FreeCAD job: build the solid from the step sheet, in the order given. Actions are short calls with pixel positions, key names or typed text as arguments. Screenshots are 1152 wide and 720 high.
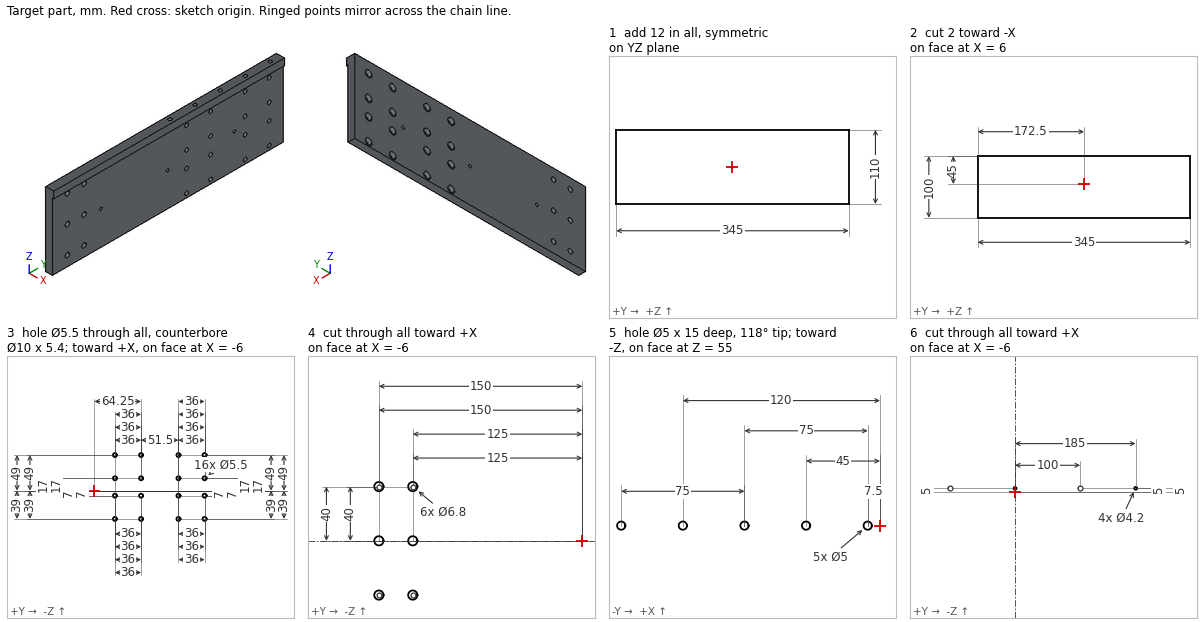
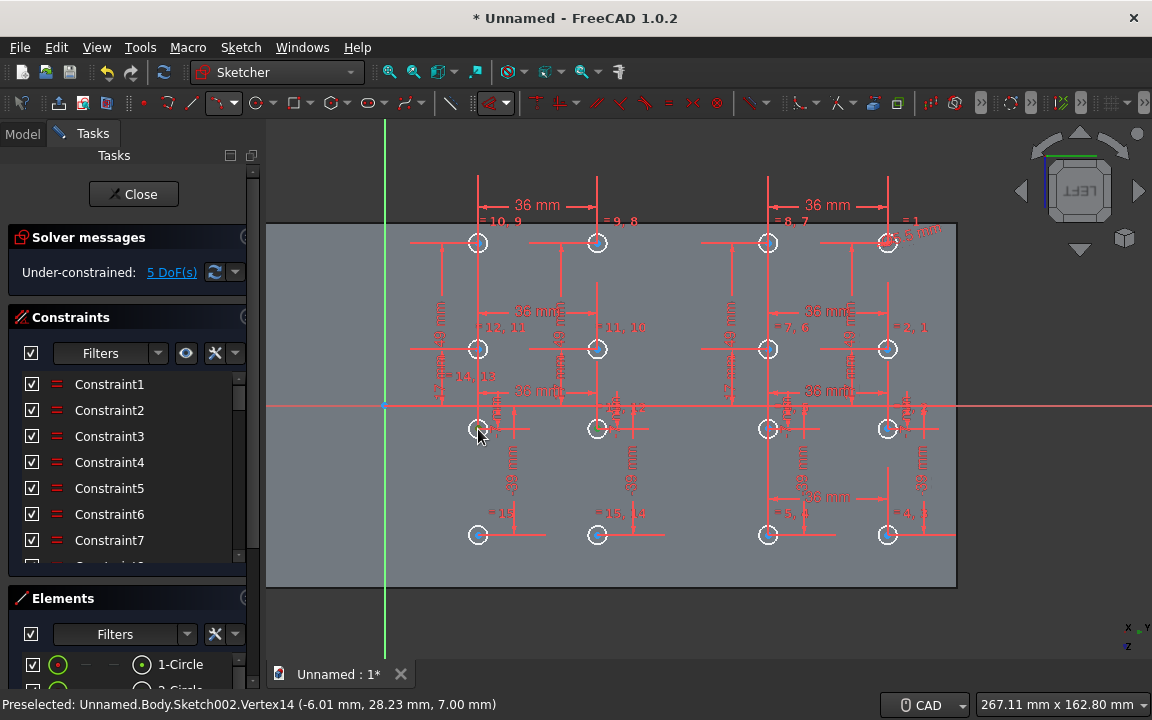
click(508, 104)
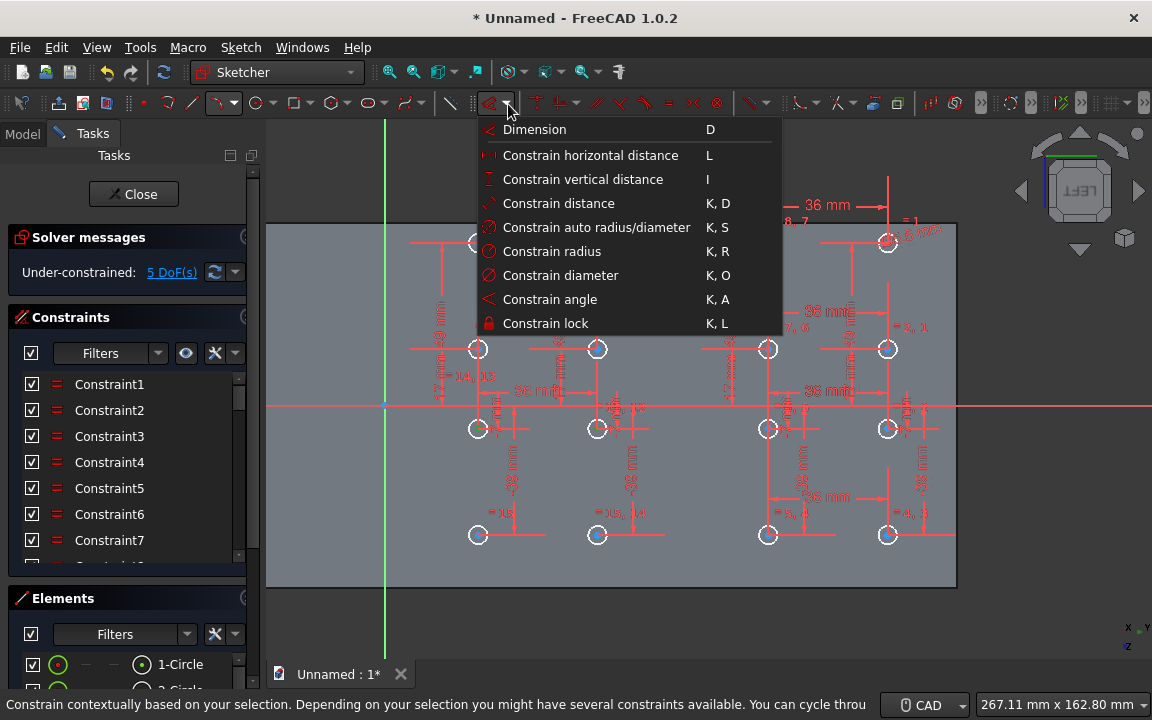
click(630, 155)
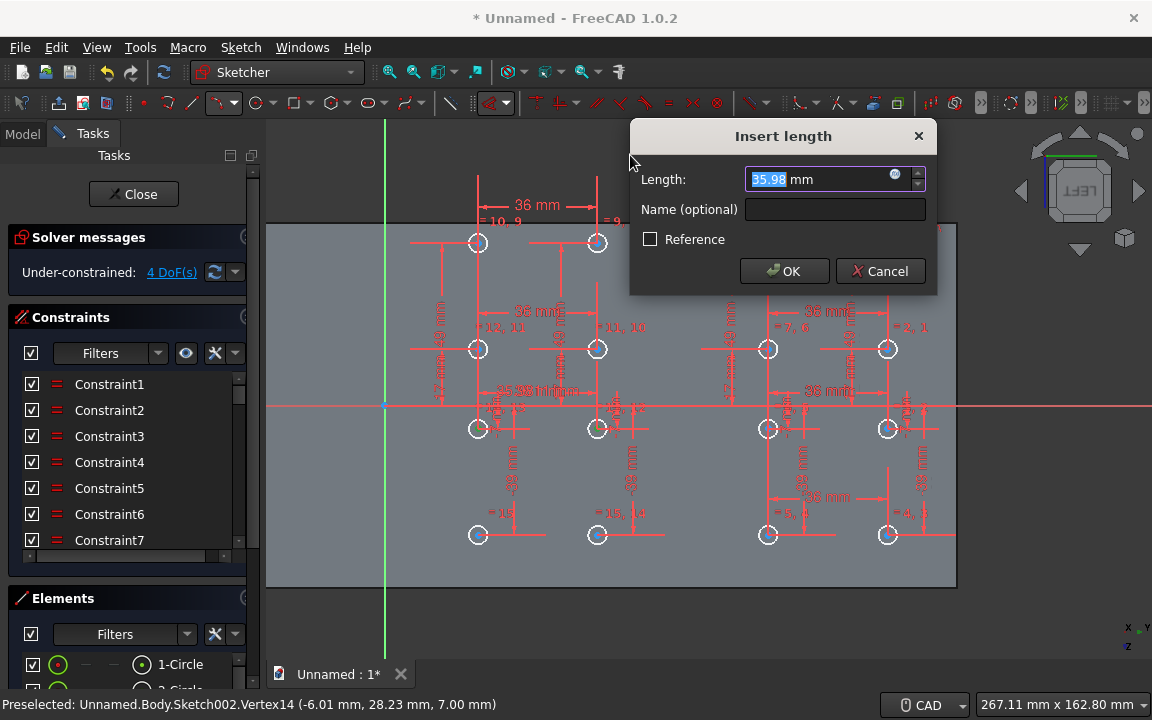
text(36)
key(Return)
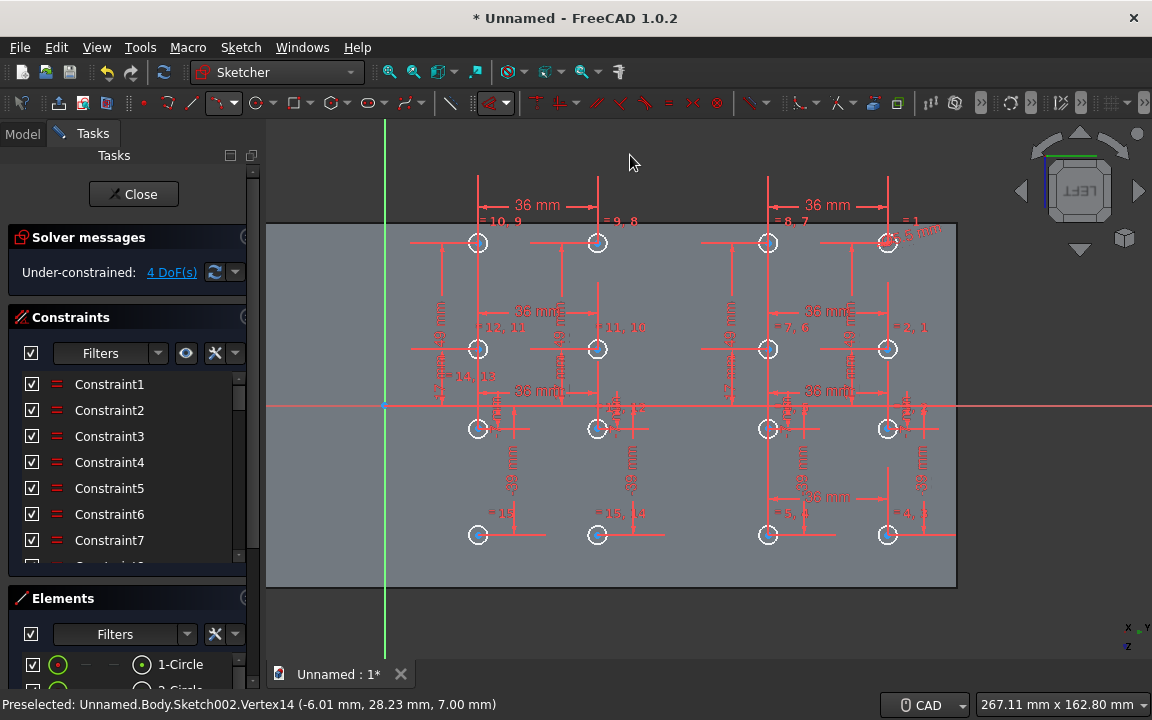
click(478, 429)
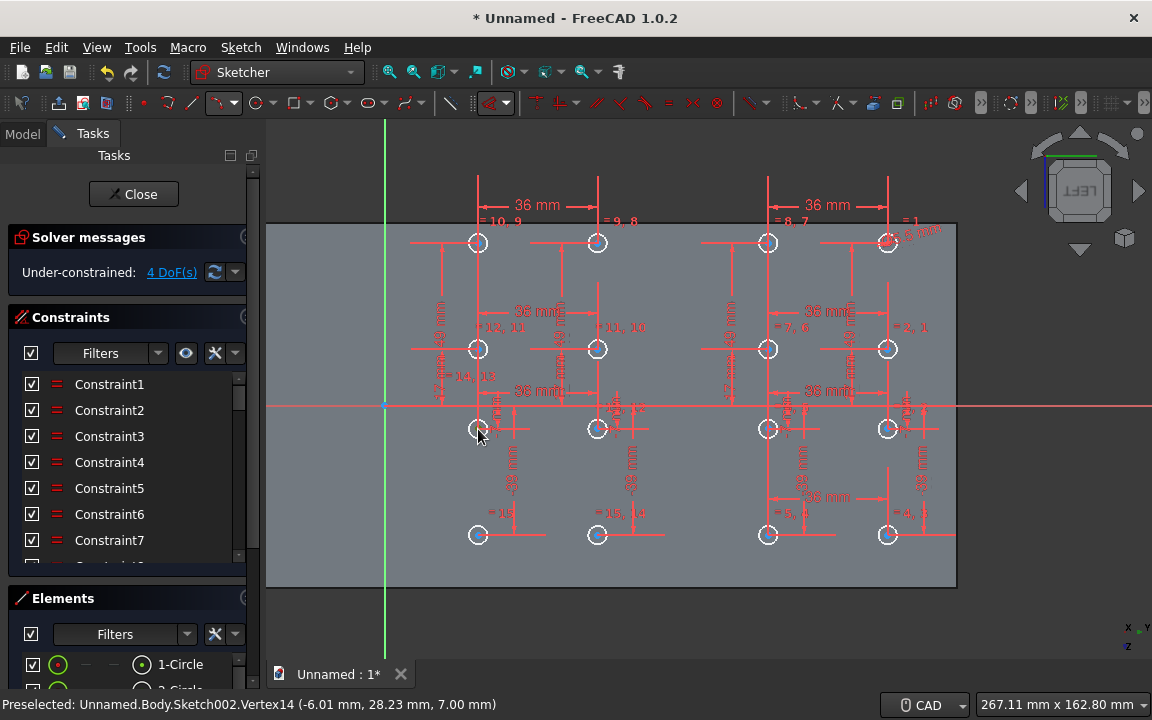
click(598, 535)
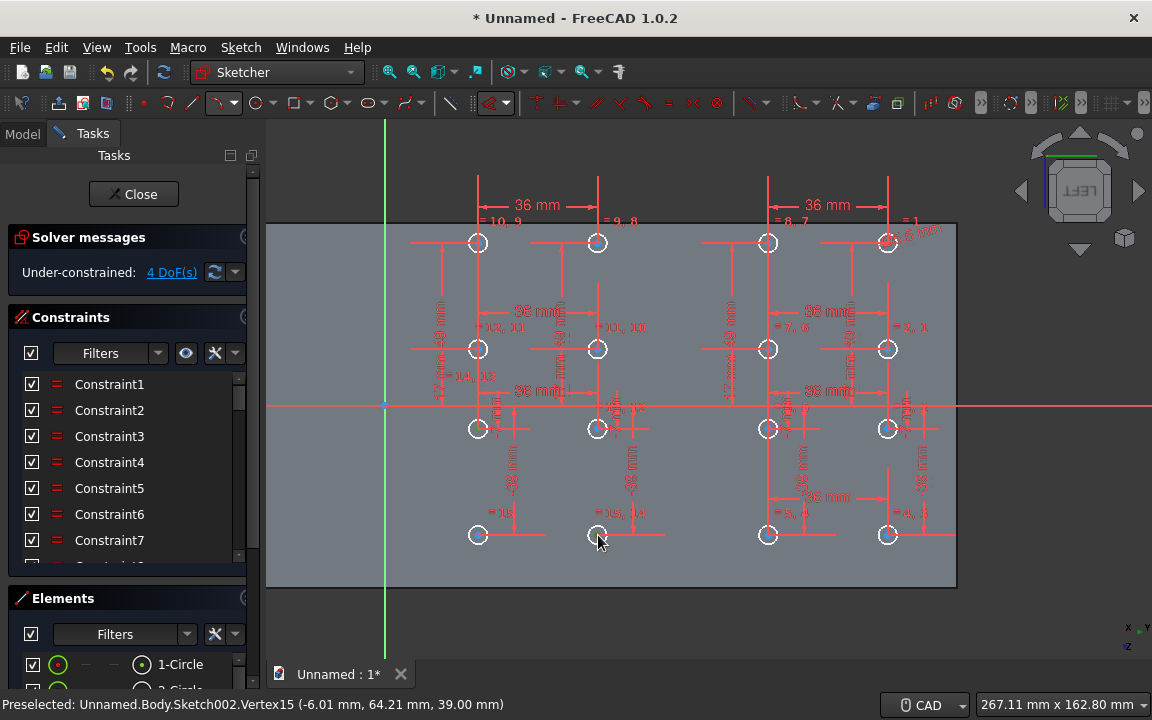
click(508, 104)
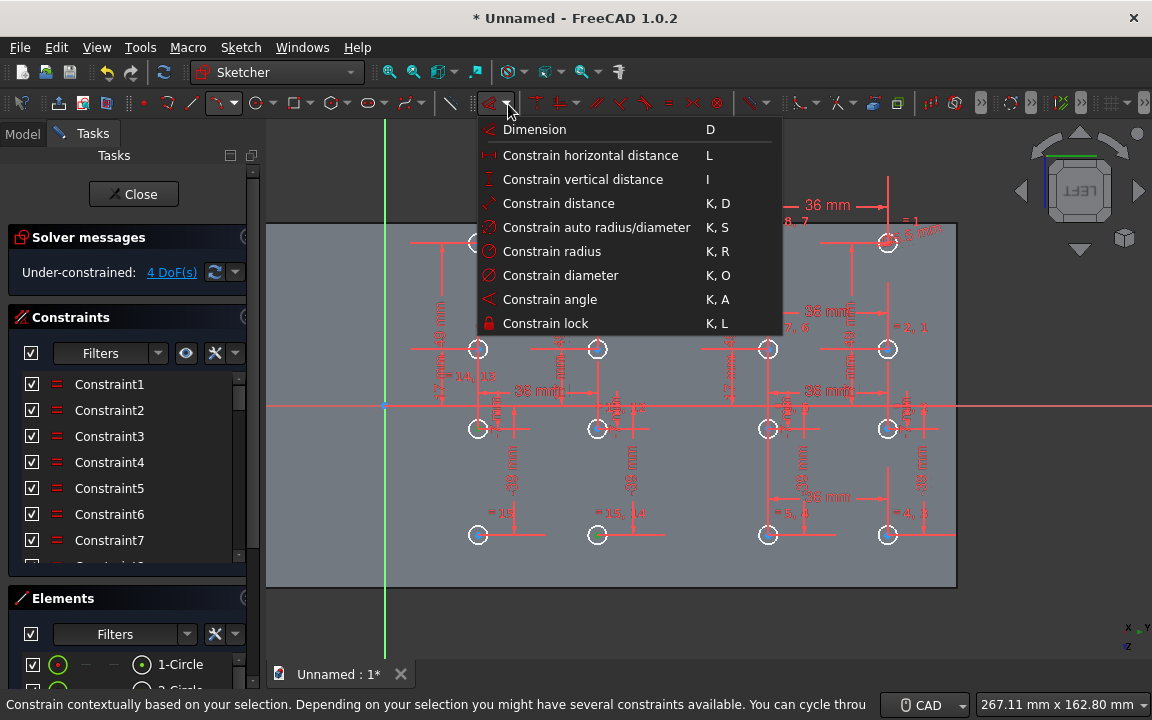
click(630, 155)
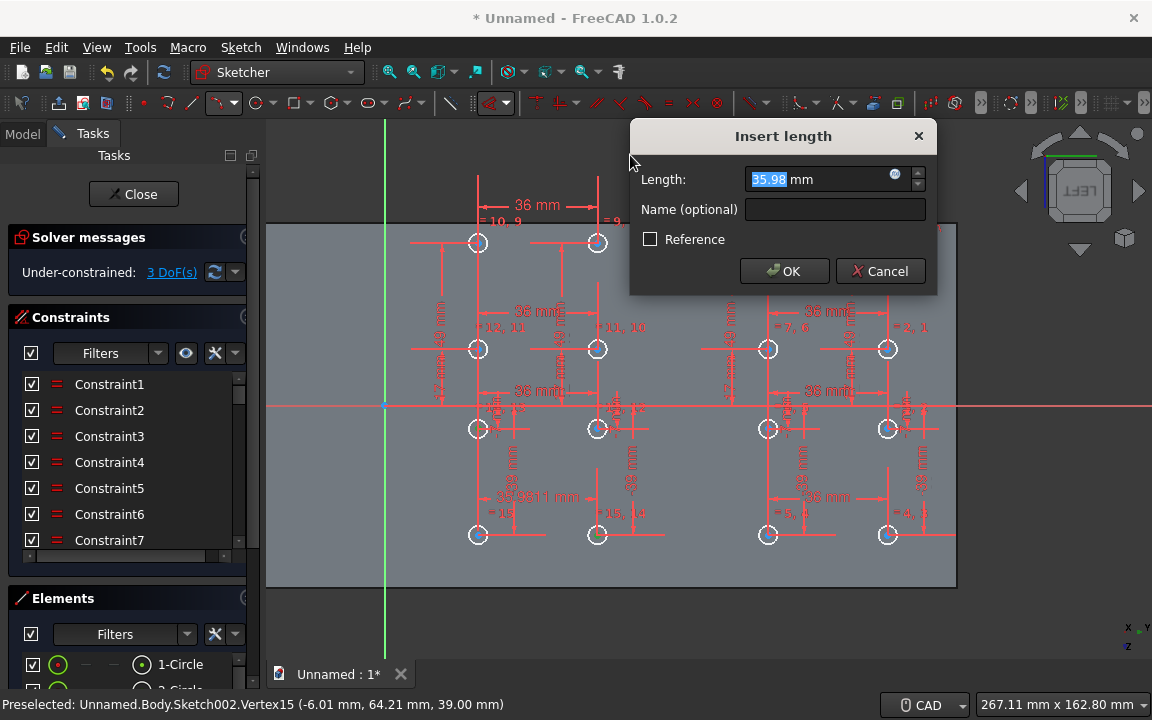
text(36)
key(Return)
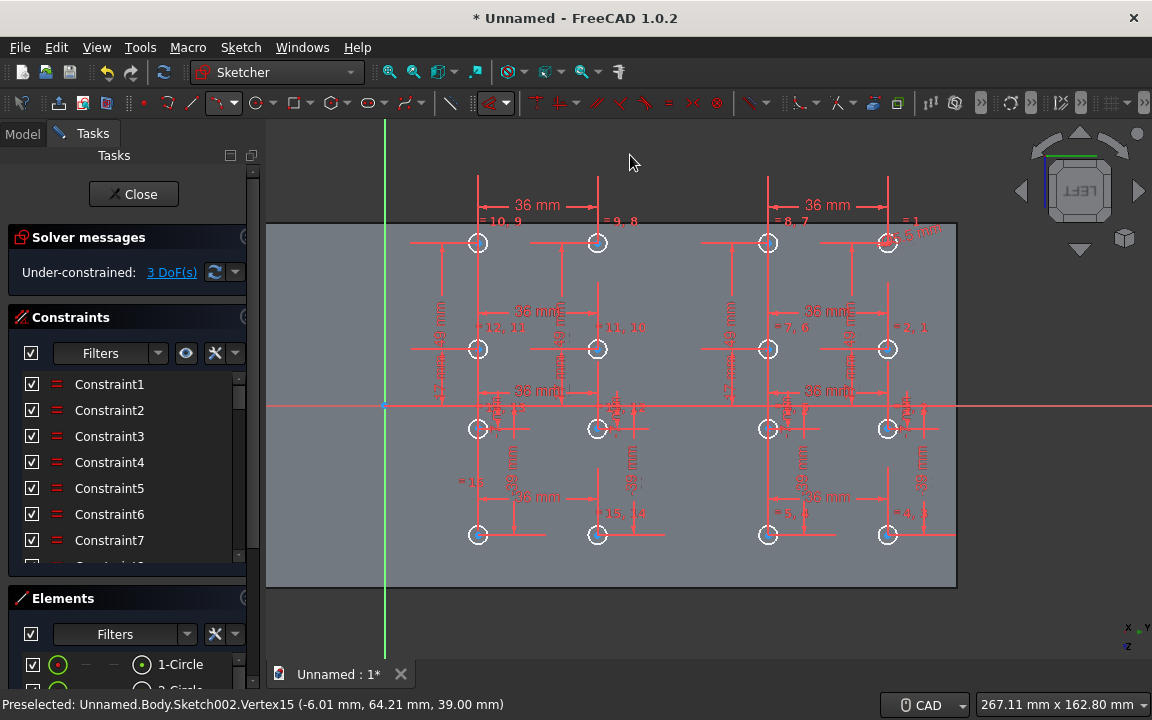
click(598, 535)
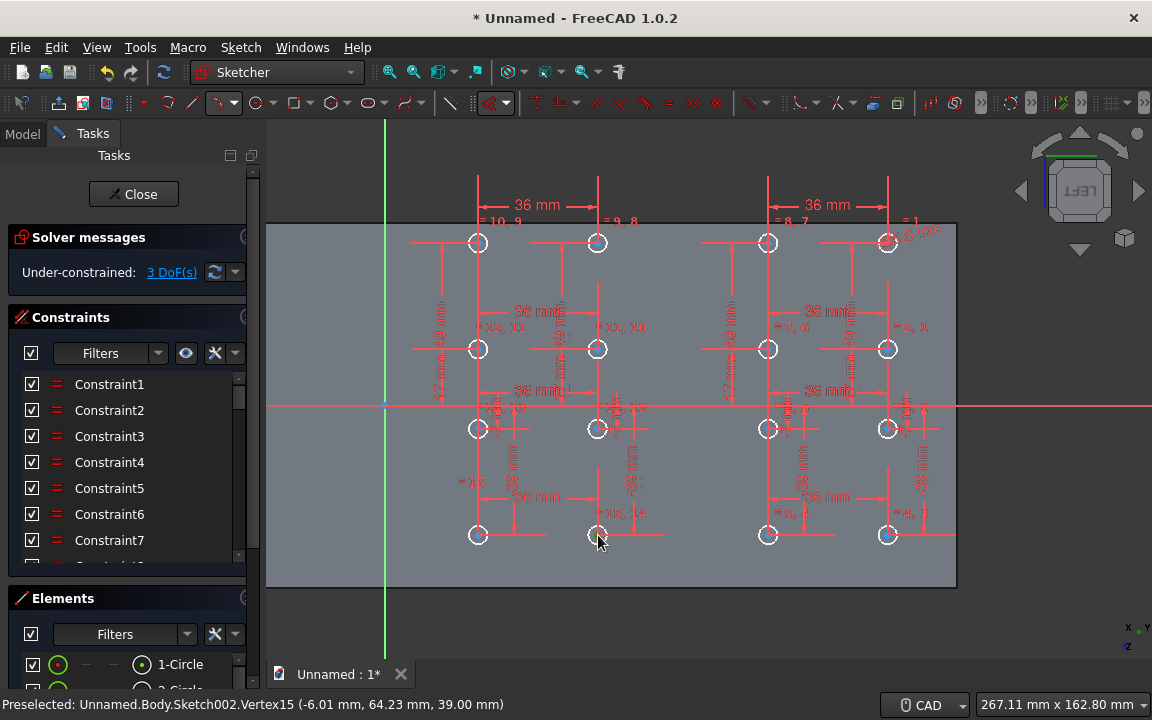
click(478, 535)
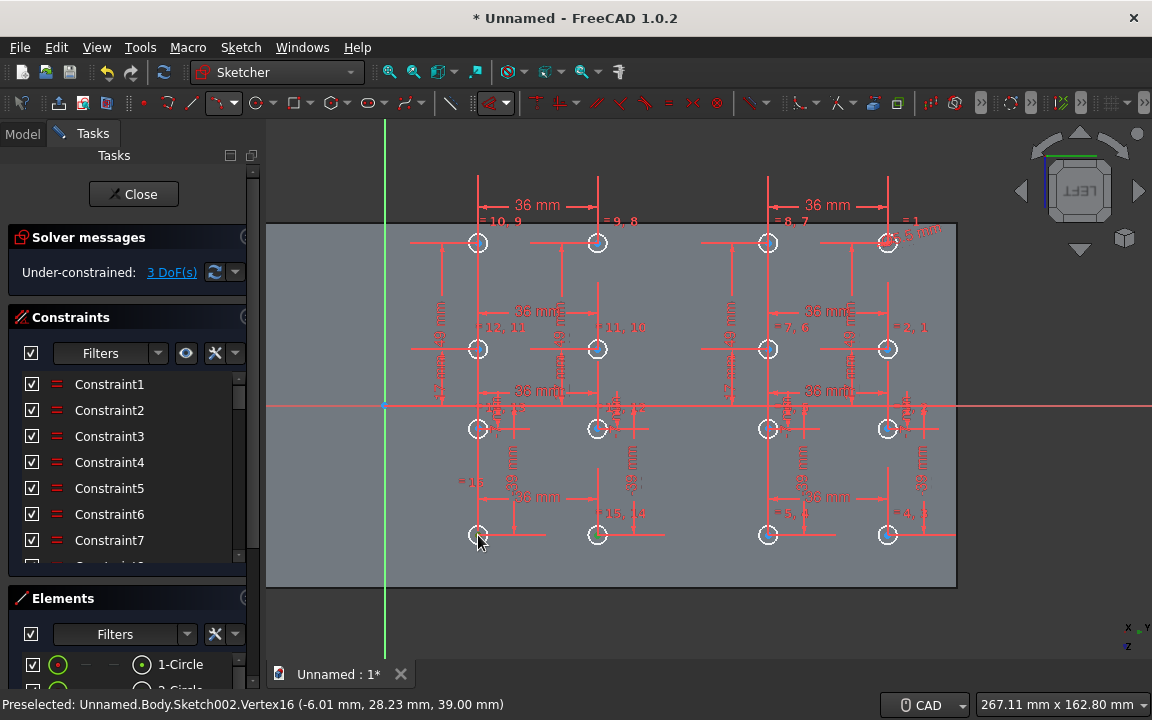
click(508, 104)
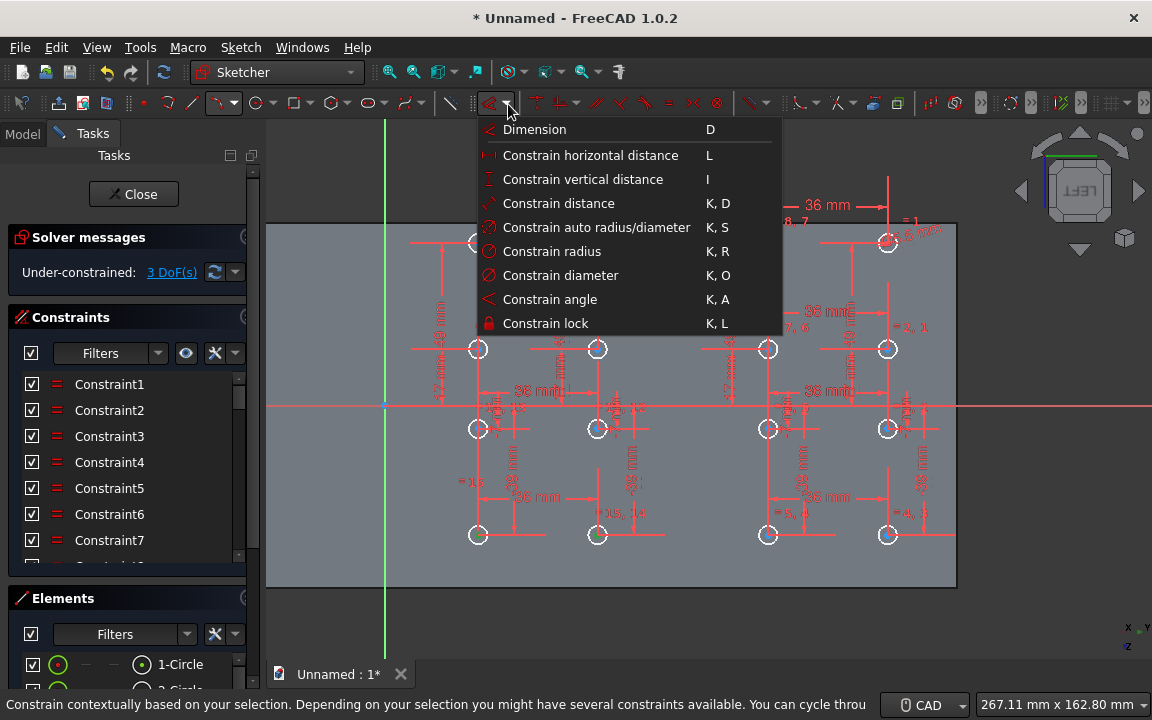
click(630, 155)